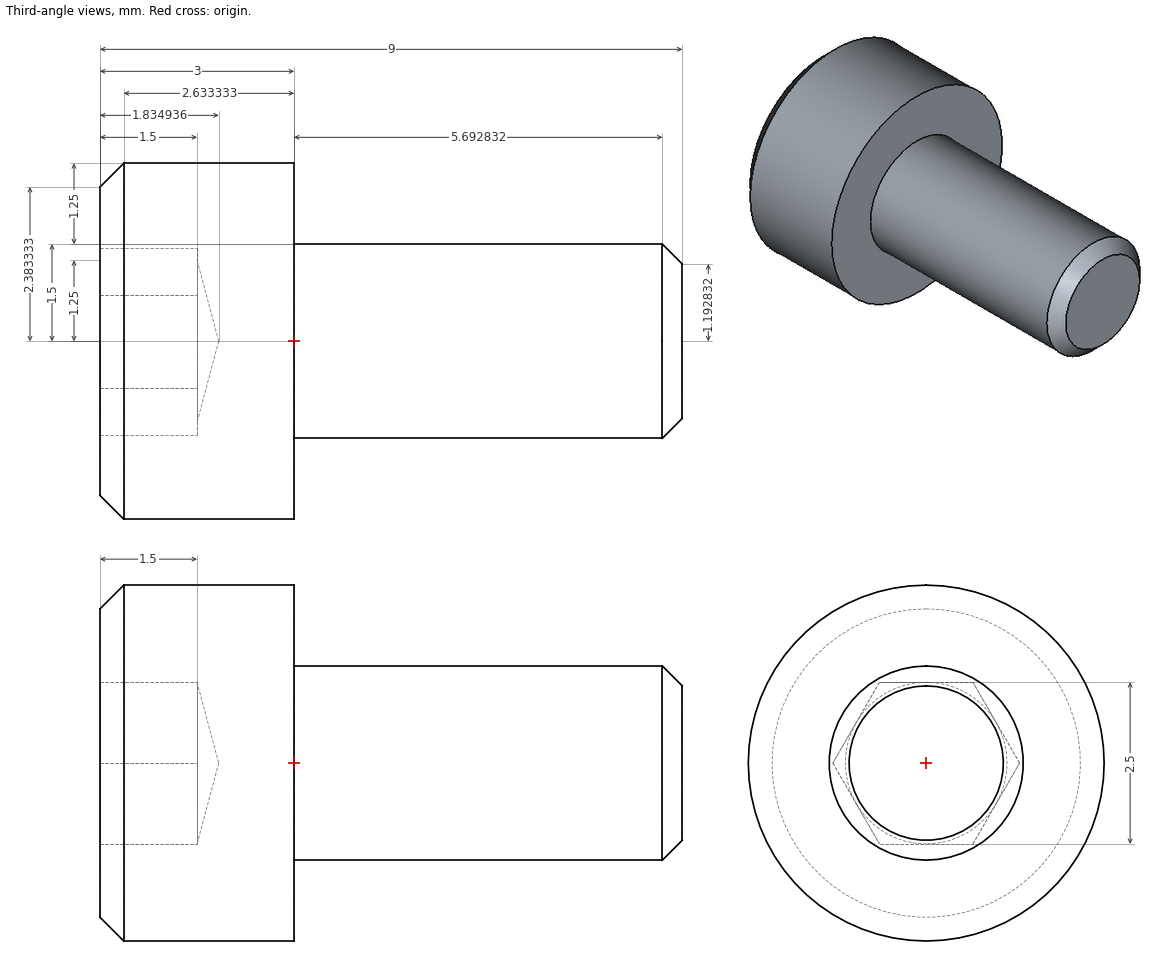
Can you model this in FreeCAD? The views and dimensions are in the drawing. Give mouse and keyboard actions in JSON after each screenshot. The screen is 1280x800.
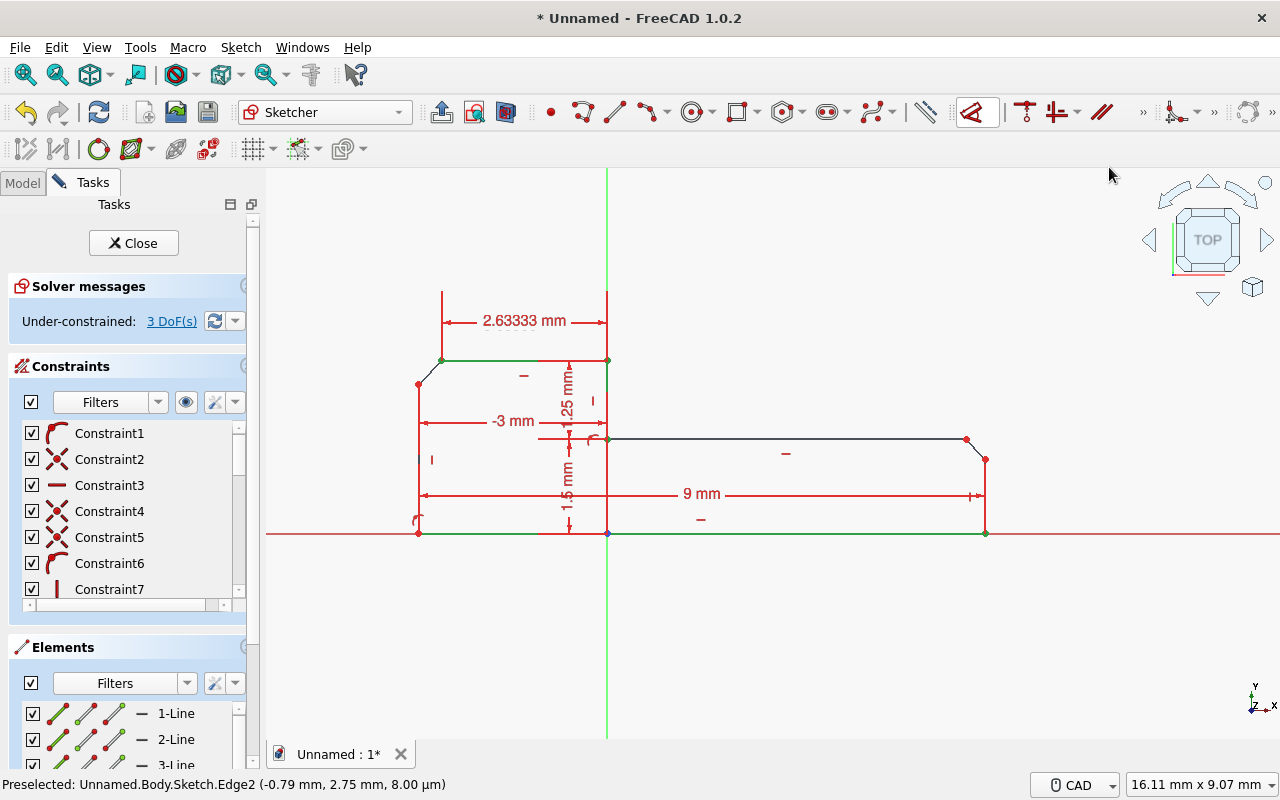
{"action": "left_click", "coordinate": [419, 430]}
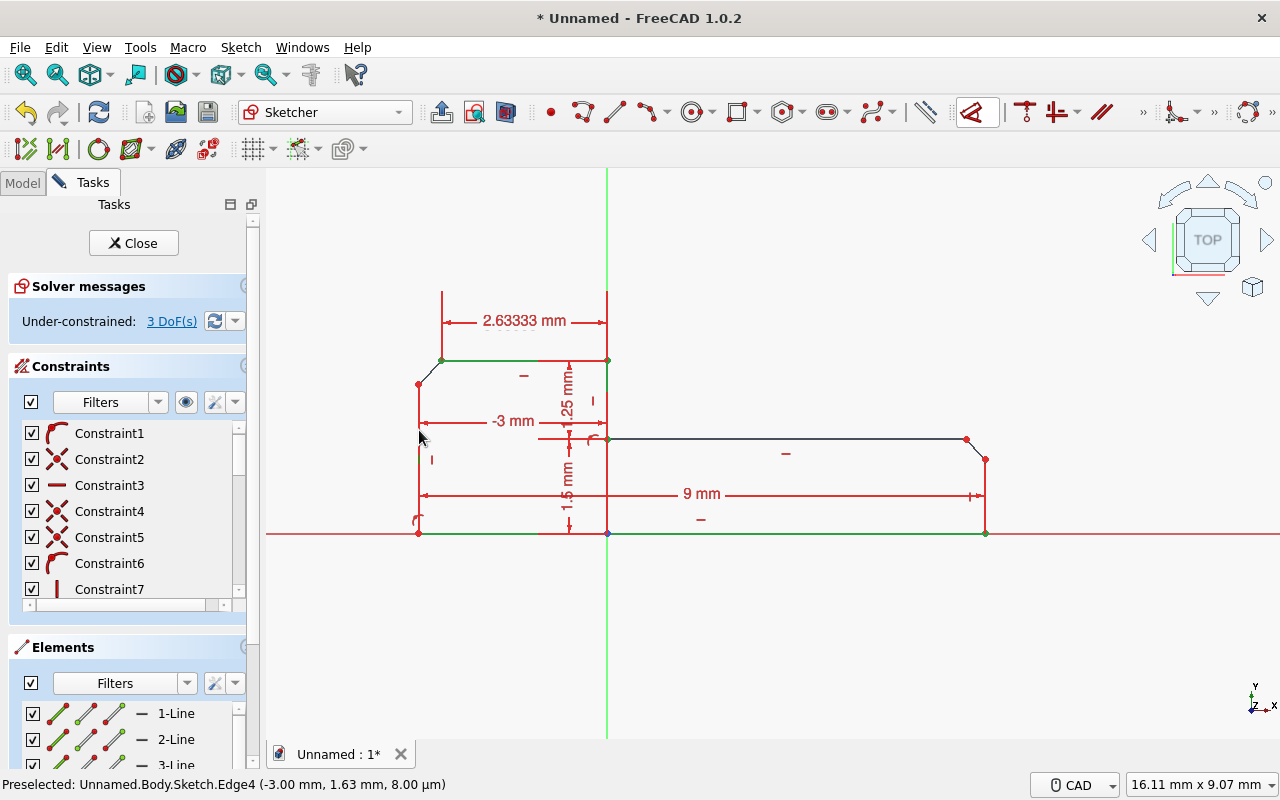
{"action": "key", "text": "i"}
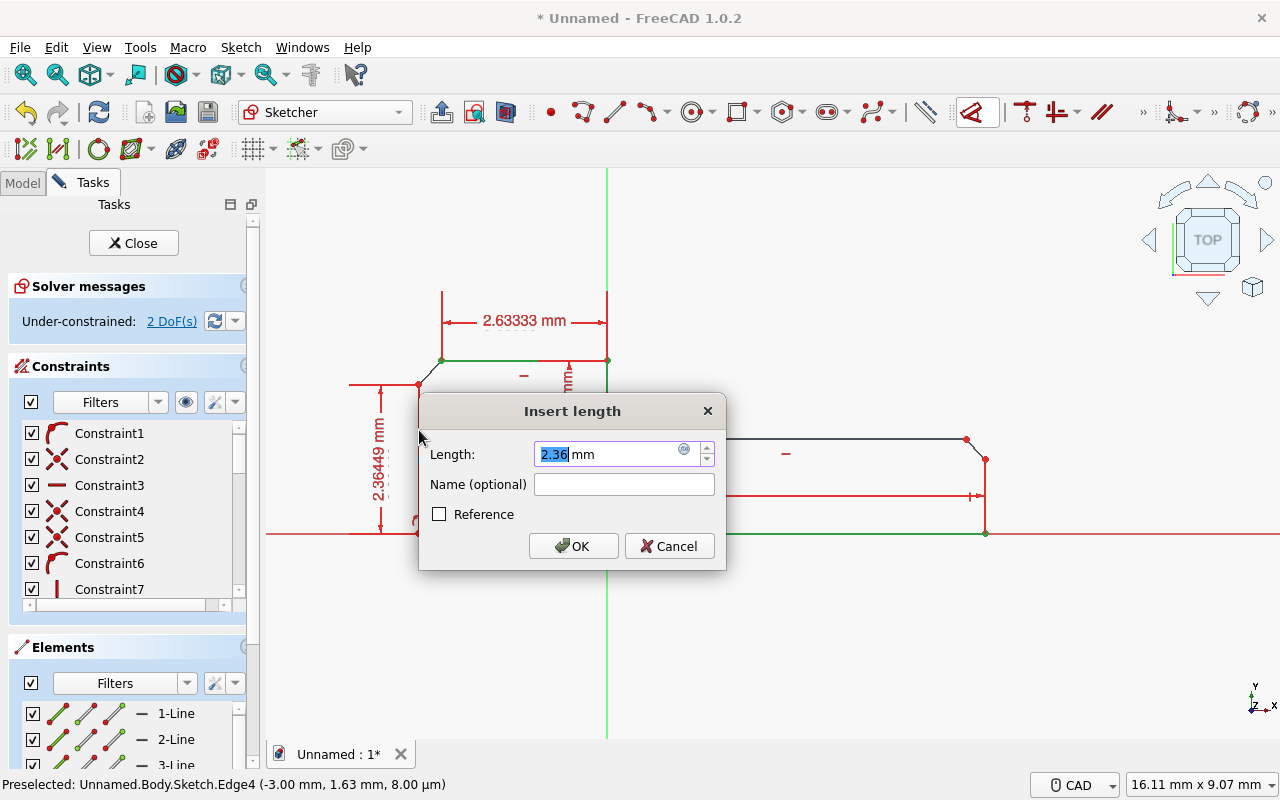
{"action": "type", "text": "2.383333"}
{"action": "key", "text": "Return"}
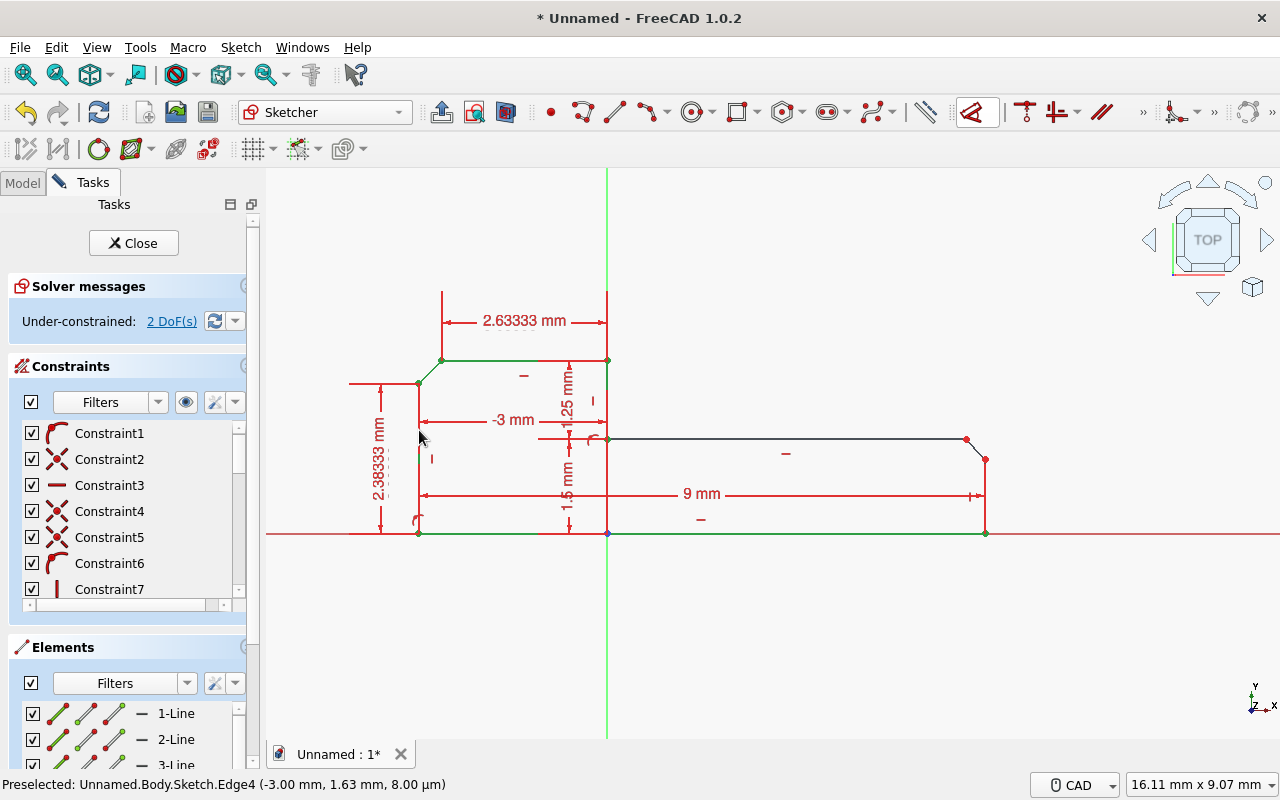
{"action": "left_click", "coordinate": [985, 512]}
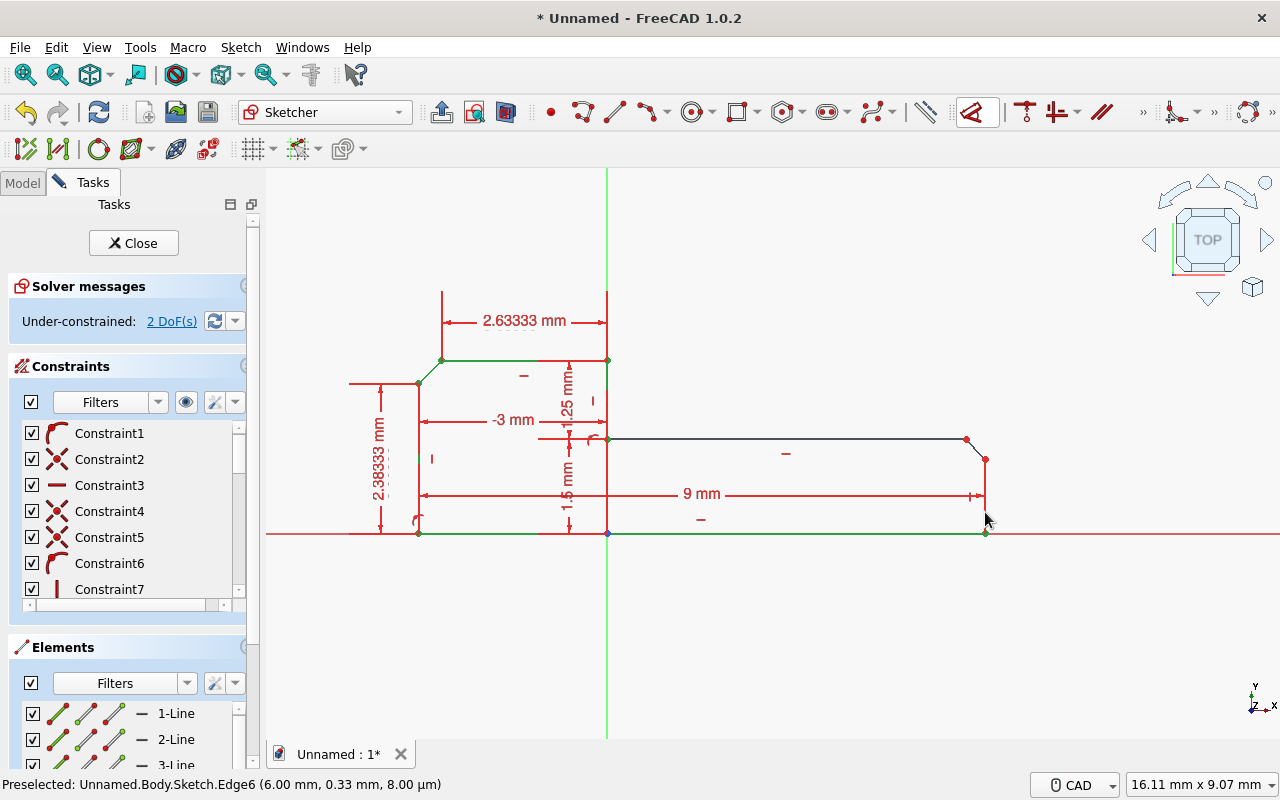
{"action": "left_click", "coordinate": [994, 112]}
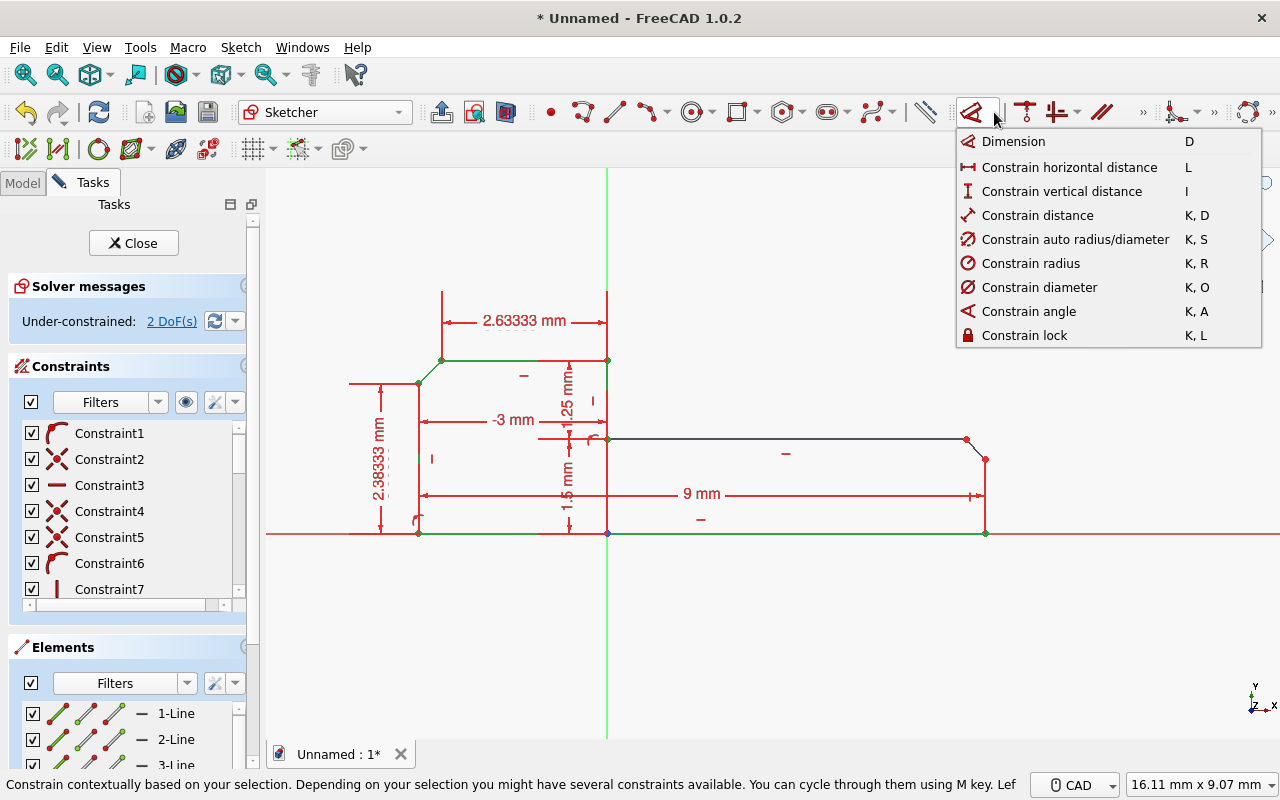
{"action": "left_click", "coordinate": [1109, 191]}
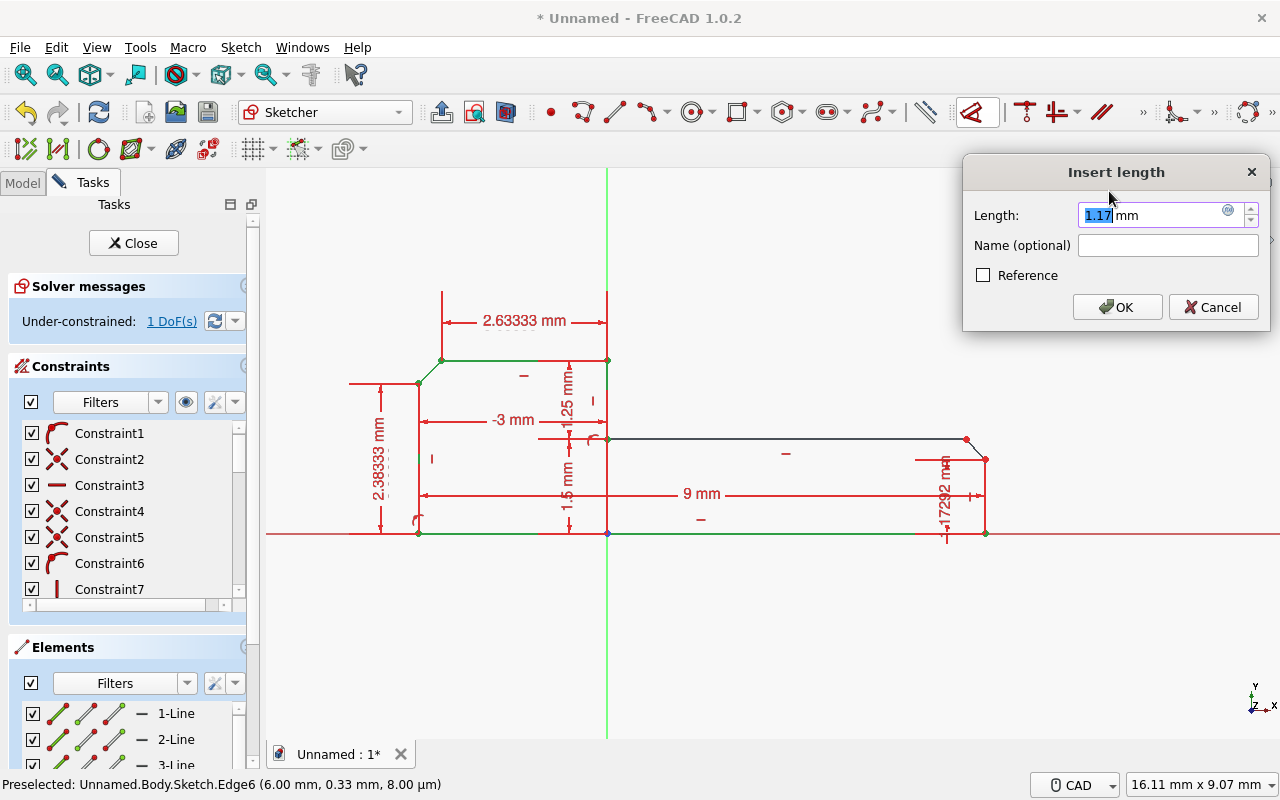
{"action": "type", "text": "1.192832"}
{"action": "key", "text": "Return"}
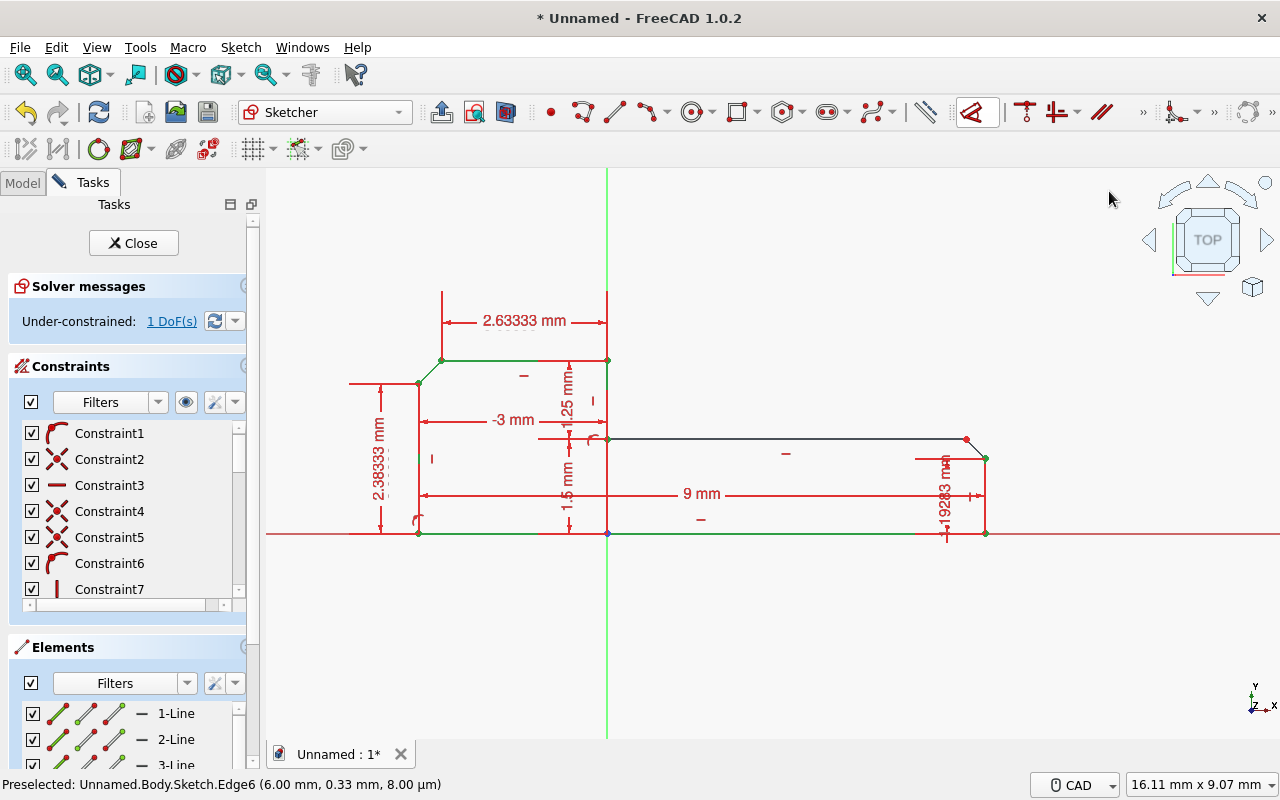
{"action": "left_click", "coordinate": [858, 439]}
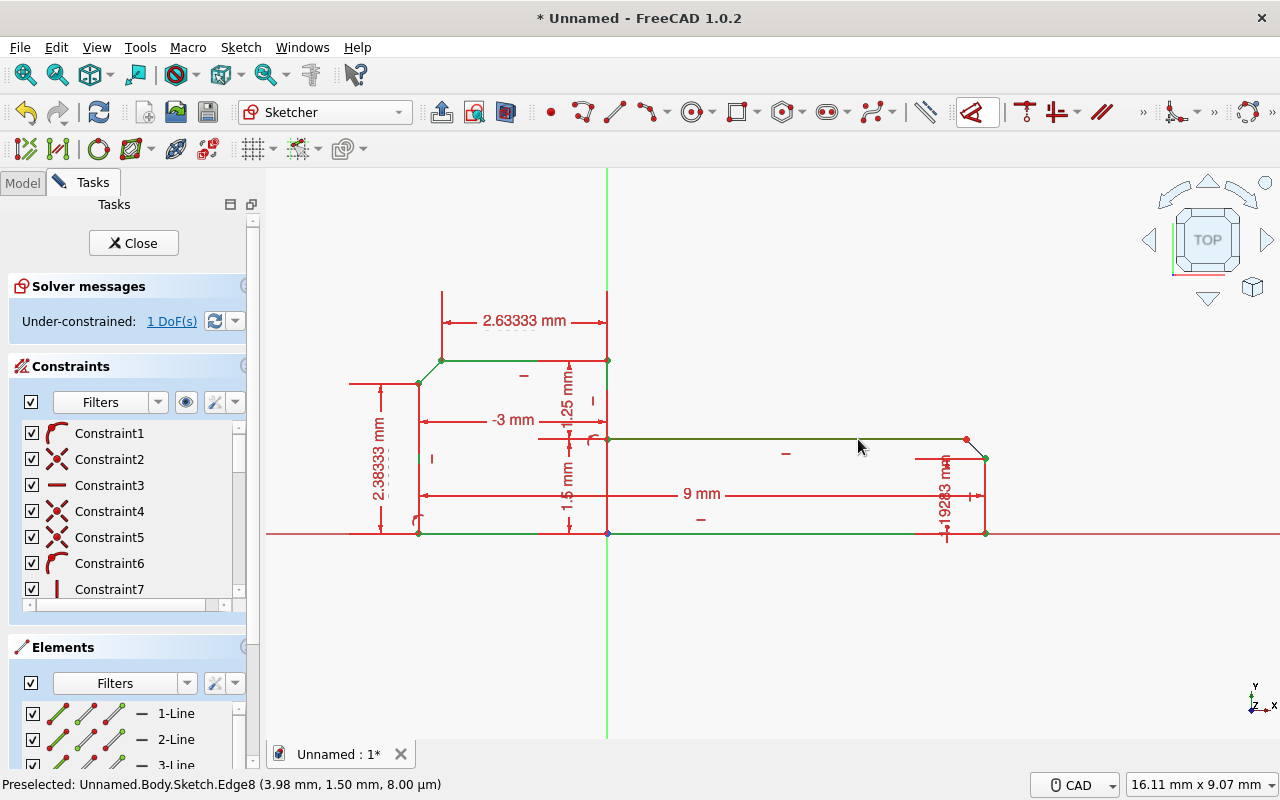
{"action": "left_click", "coordinate": [994, 112]}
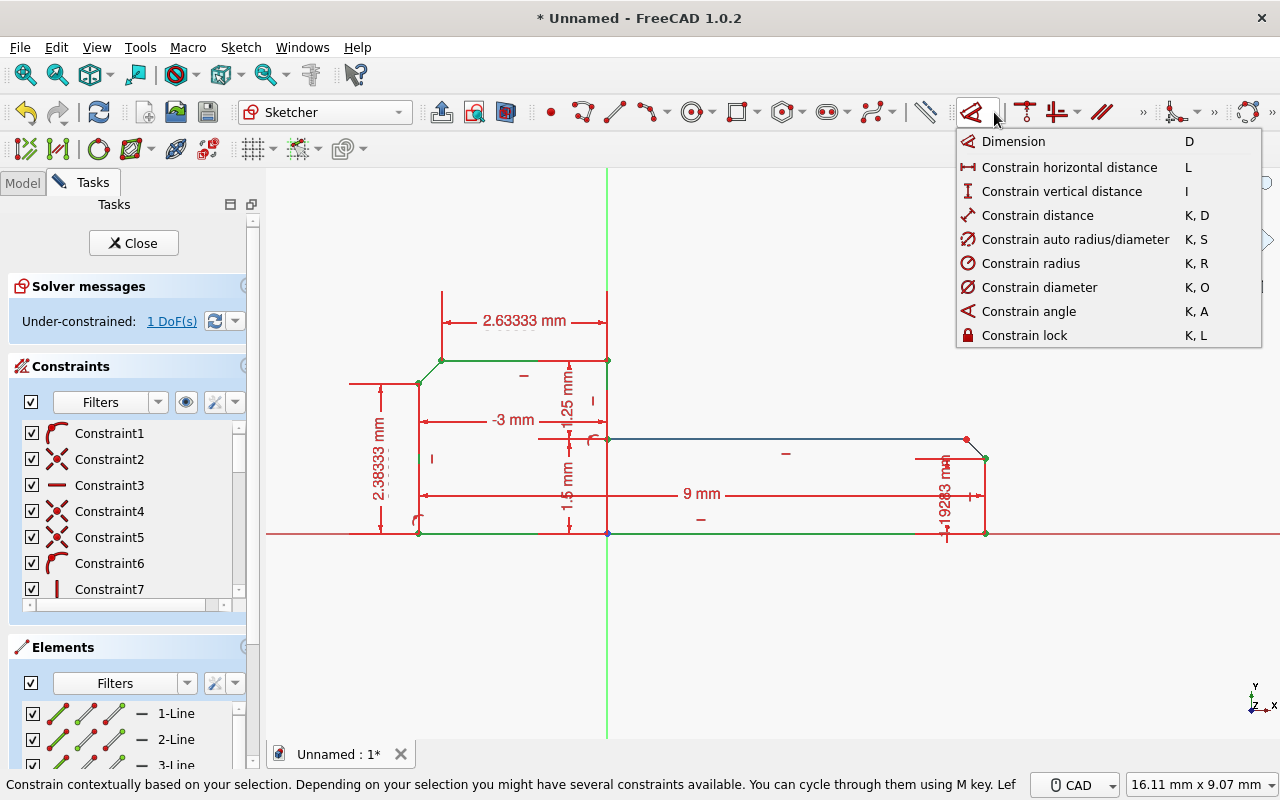
{"action": "left_click", "coordinate": [1109, 167]}